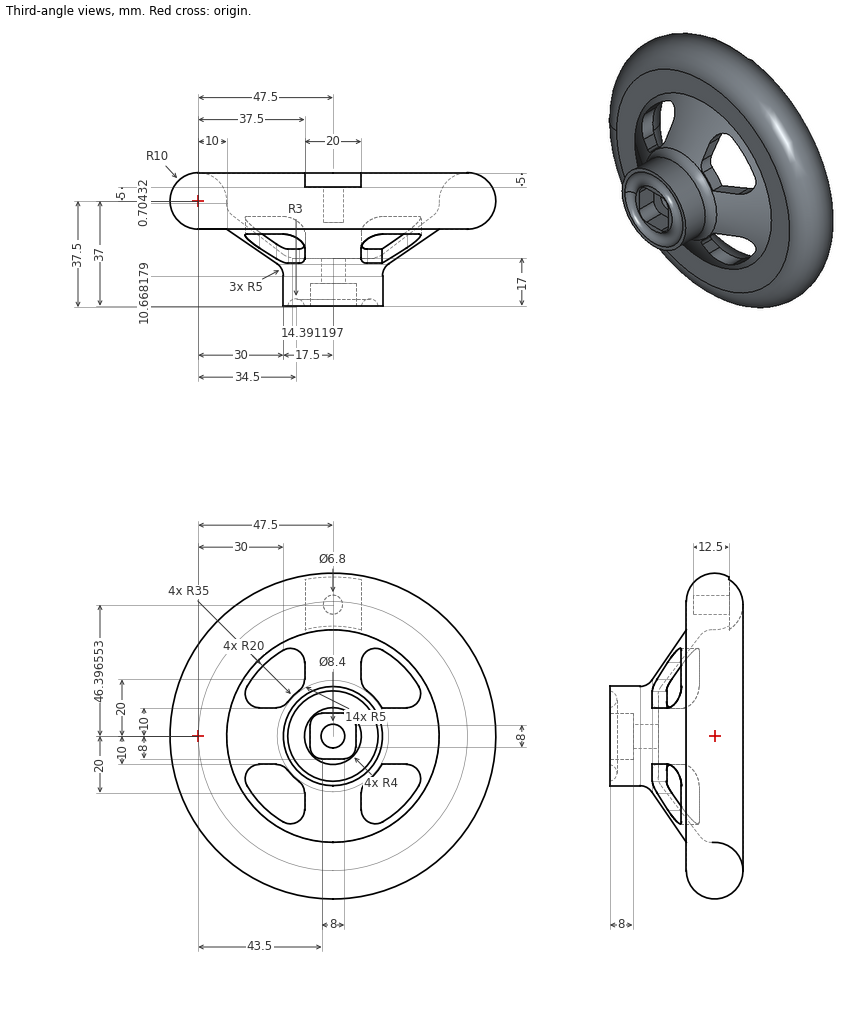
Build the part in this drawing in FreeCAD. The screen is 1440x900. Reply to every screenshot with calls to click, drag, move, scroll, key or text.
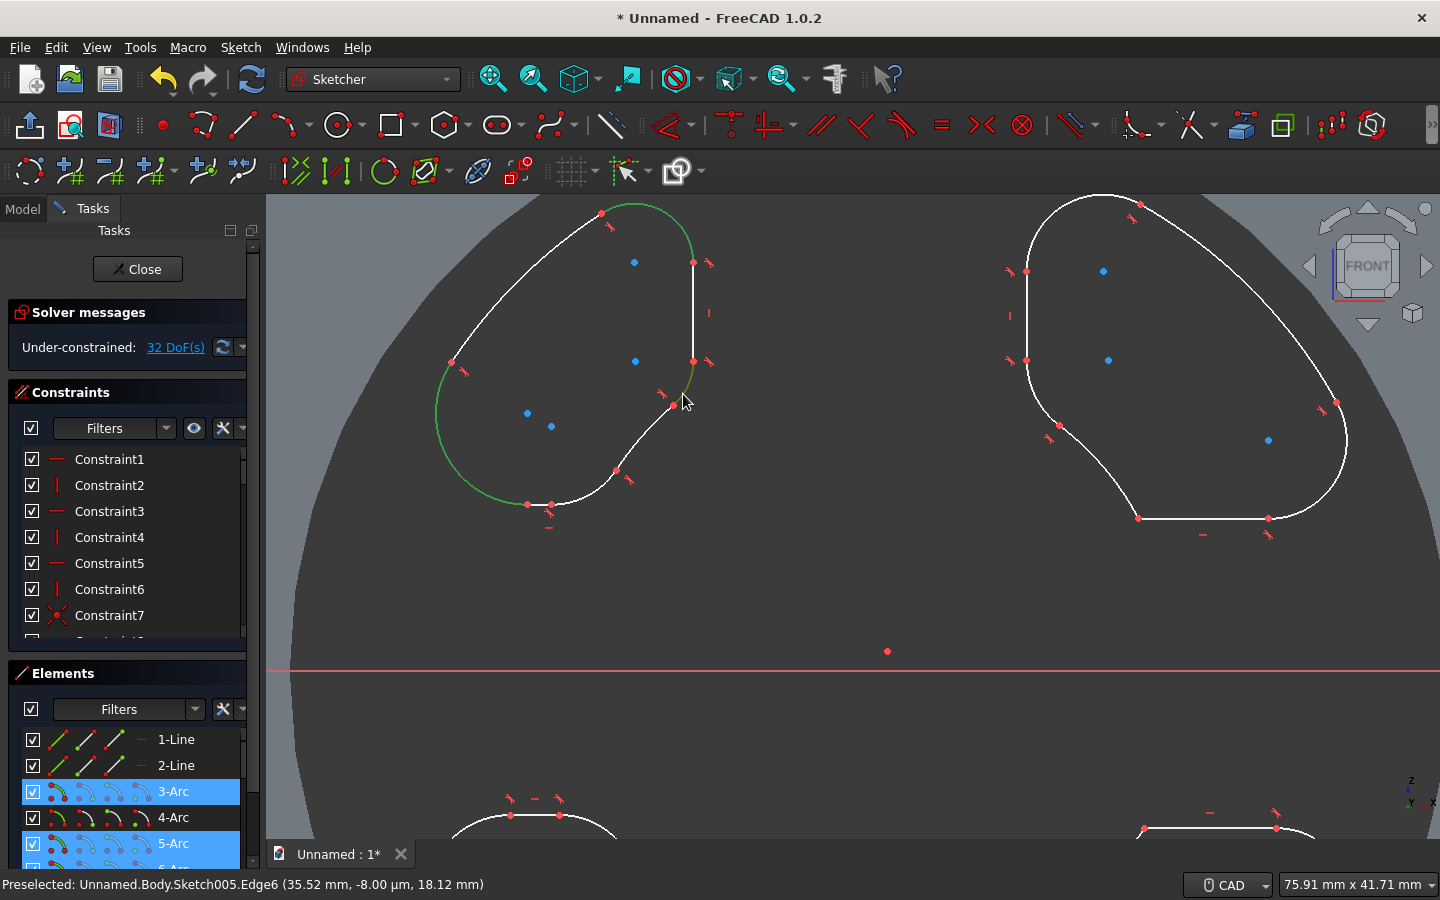
click(574, 501)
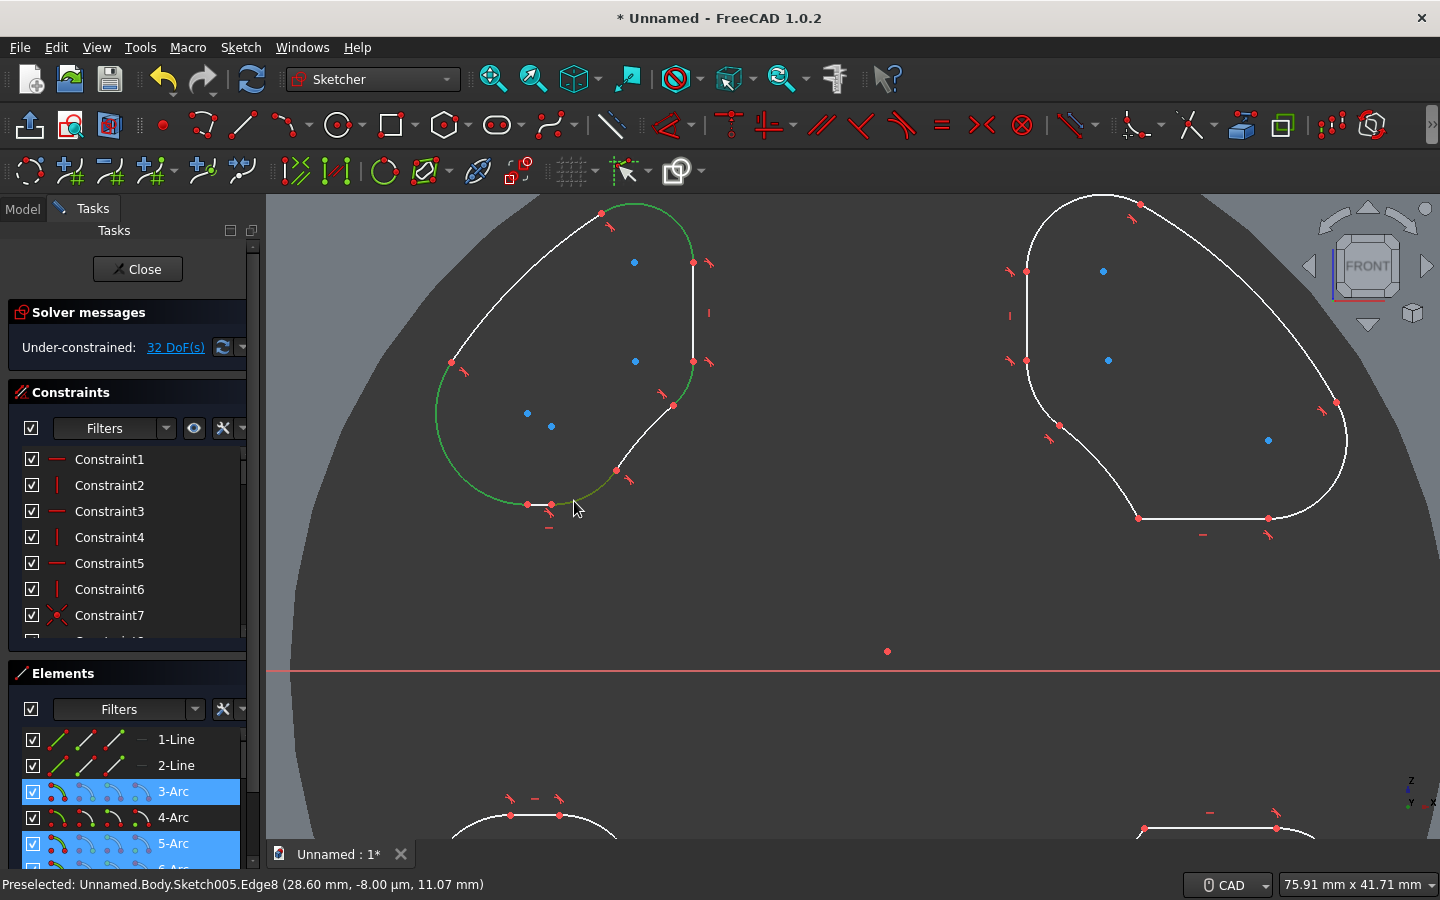
scroll(823, 390, down, 4)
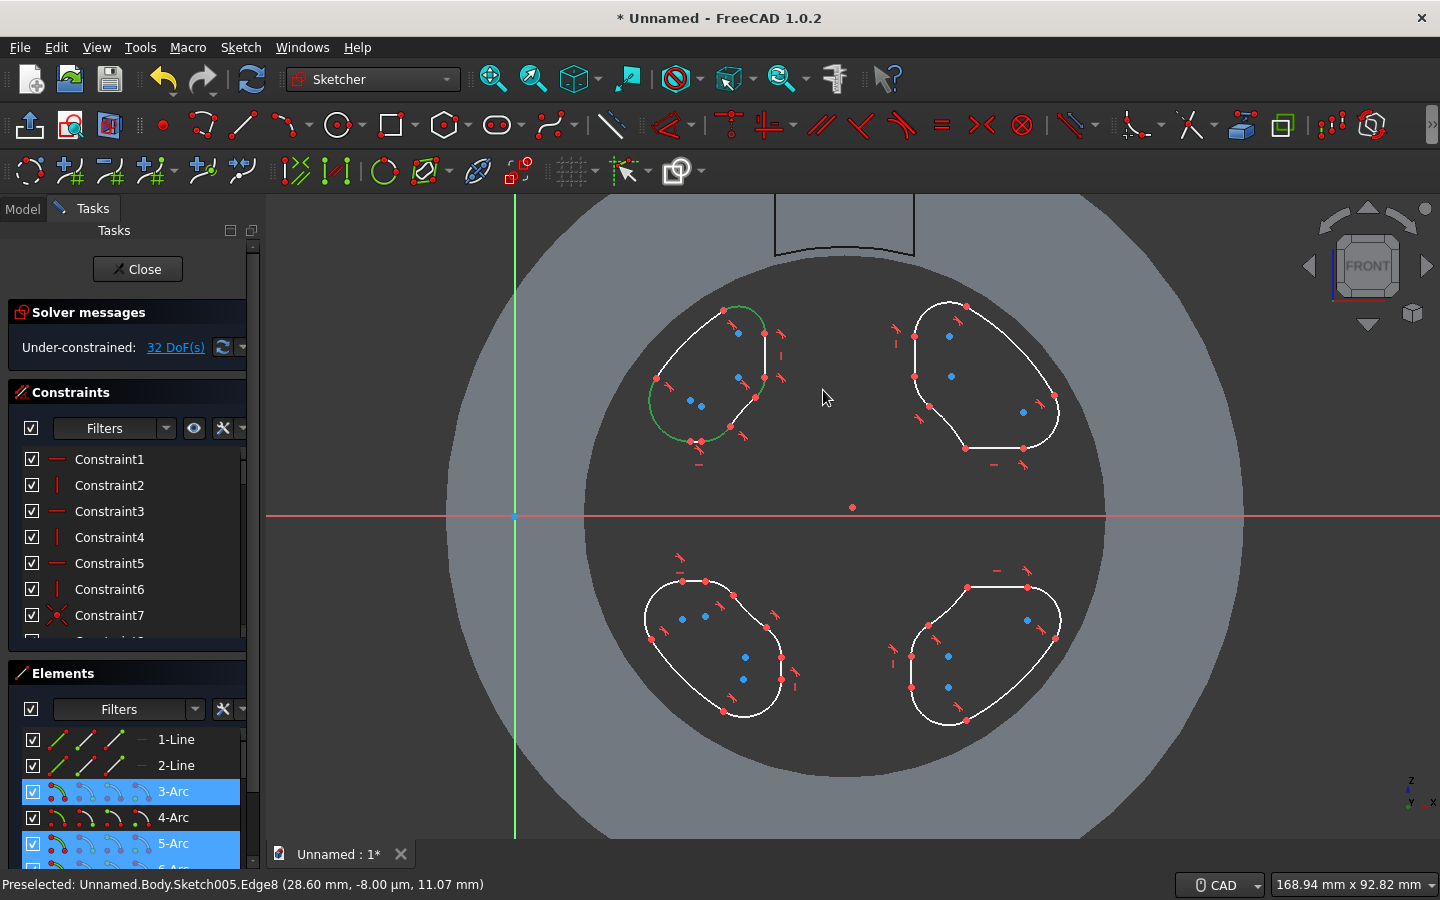
scroll(726, 588, up, 2)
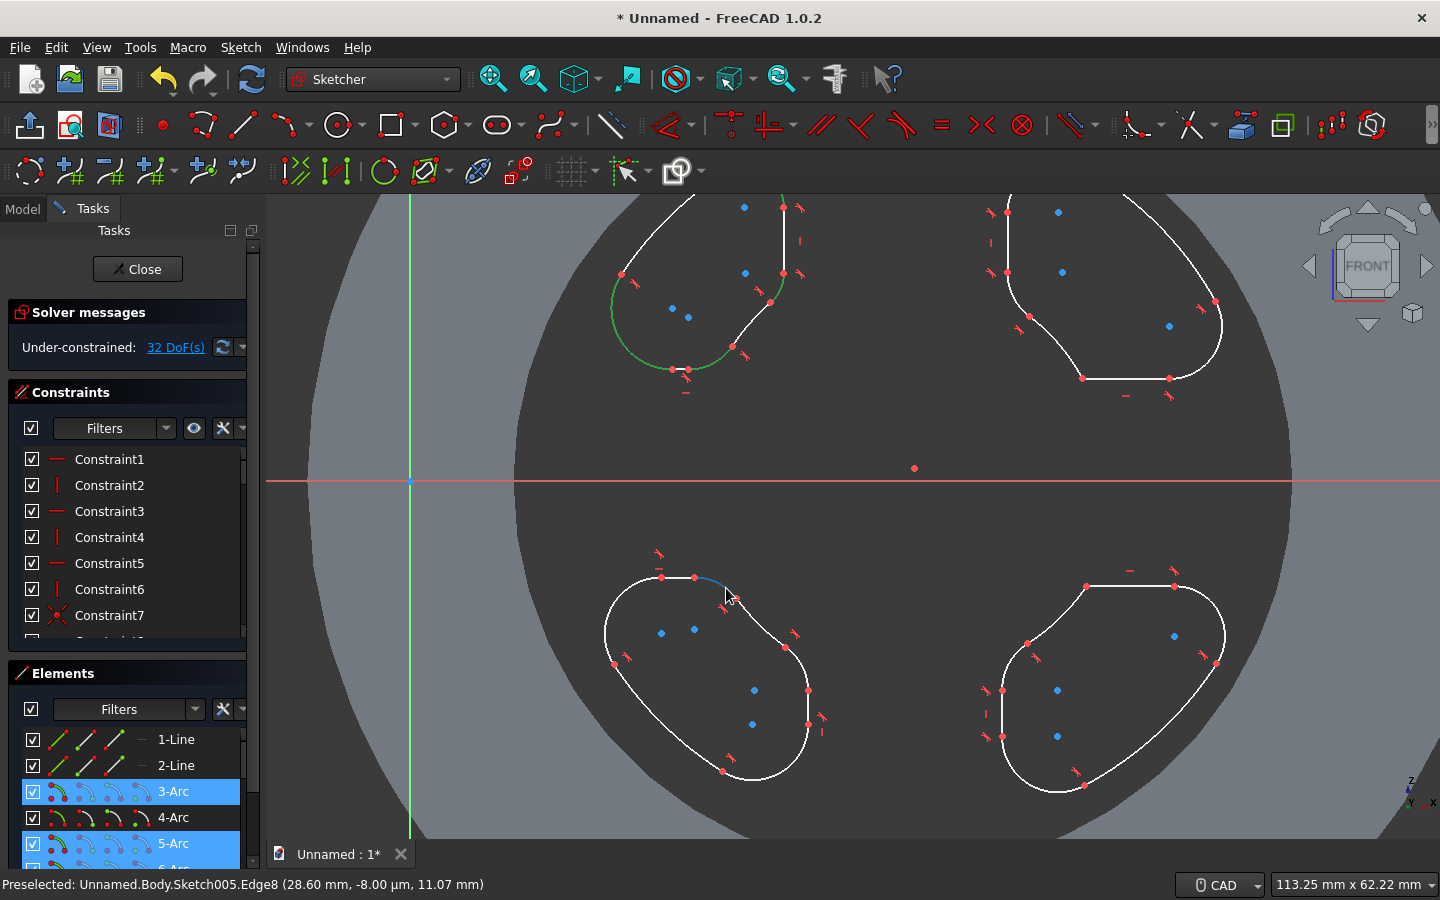
click(727, 588)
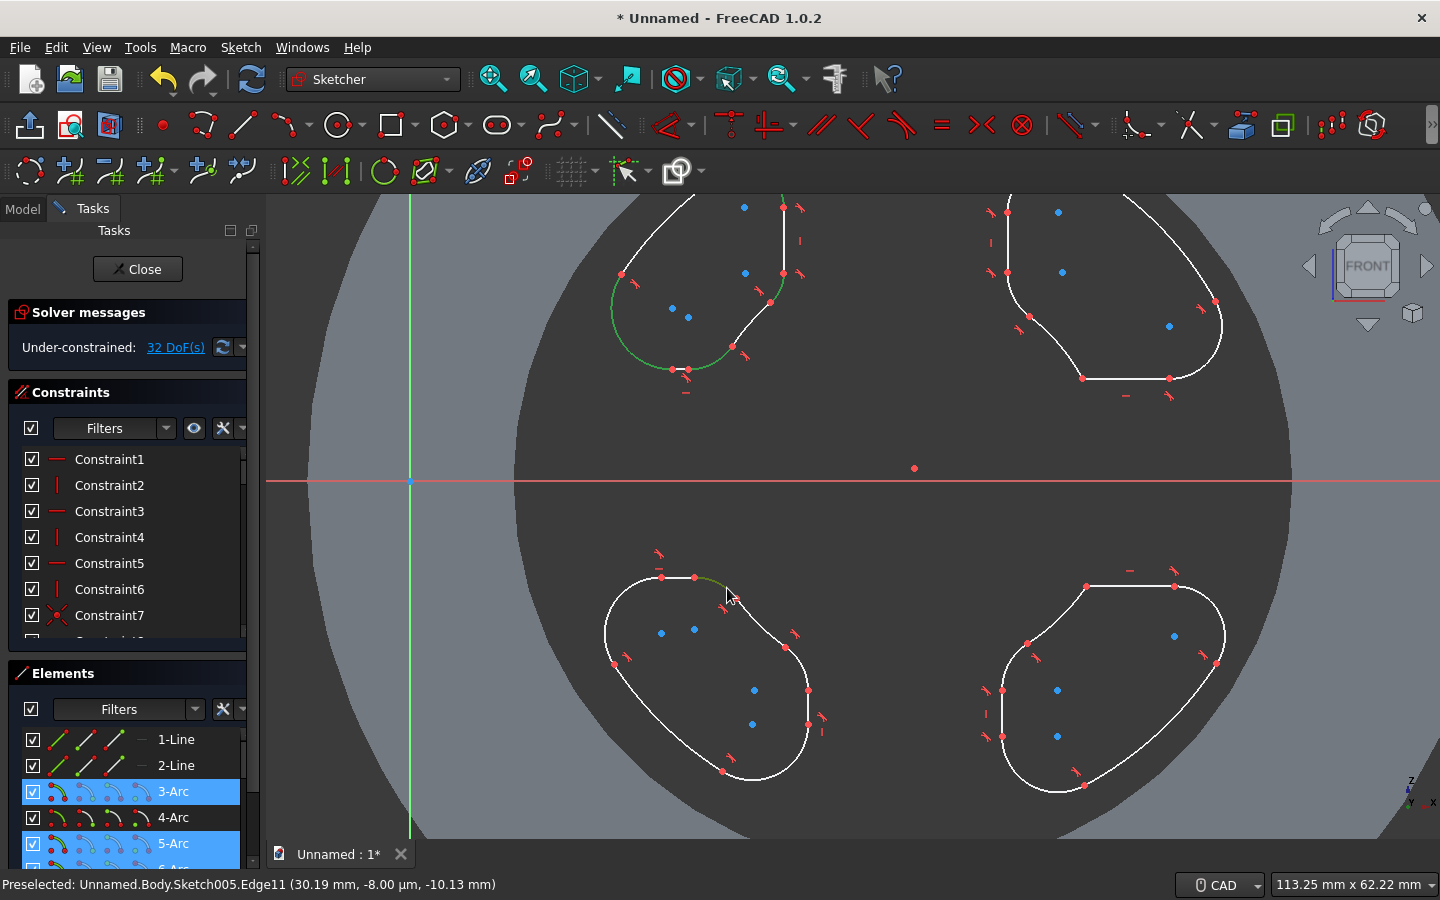
click(806, 676)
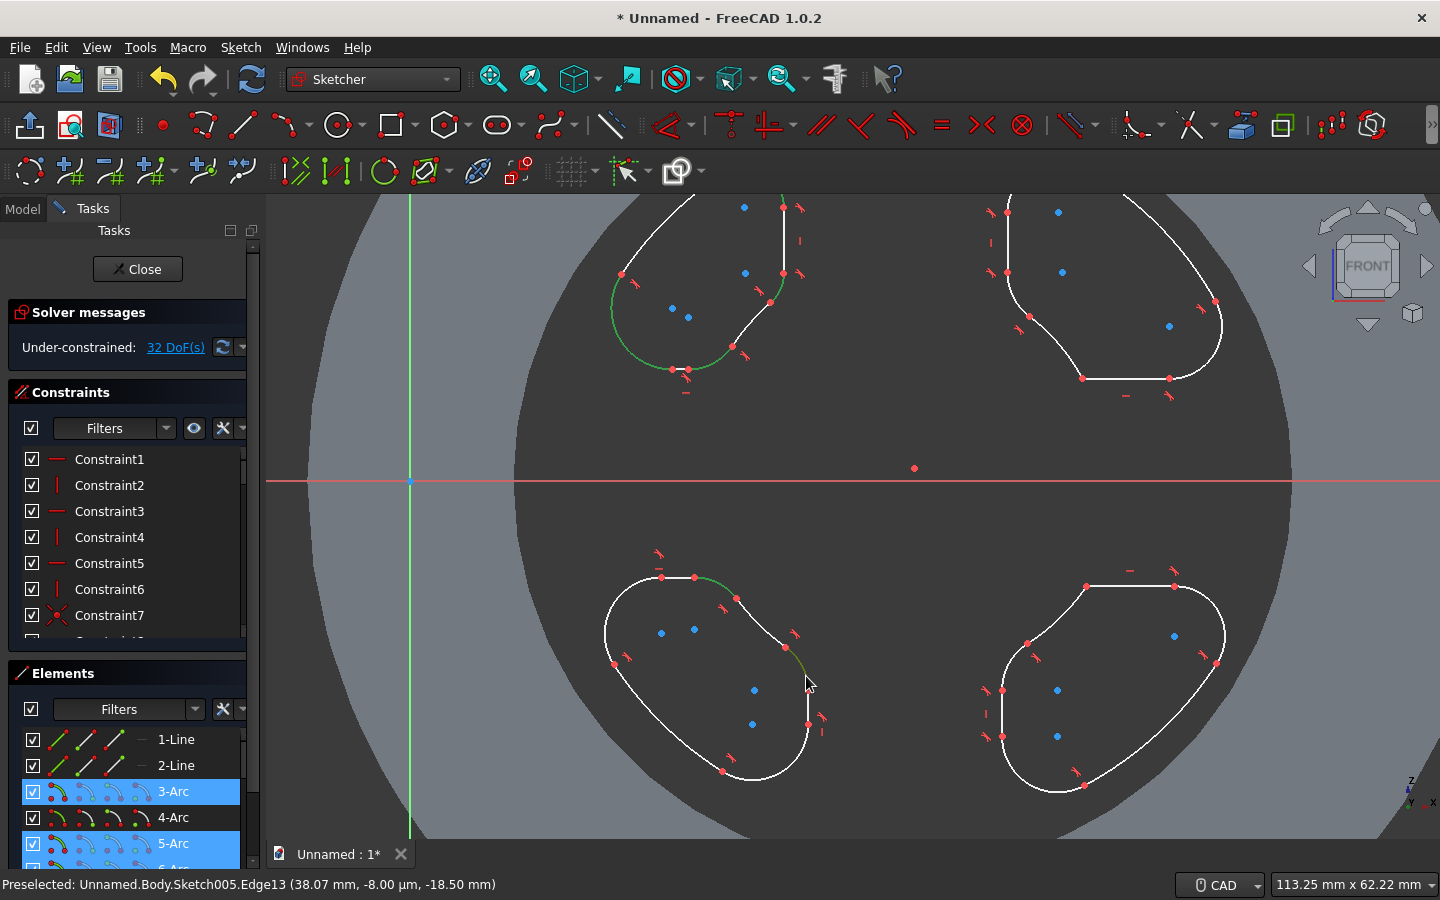
click(757, 780)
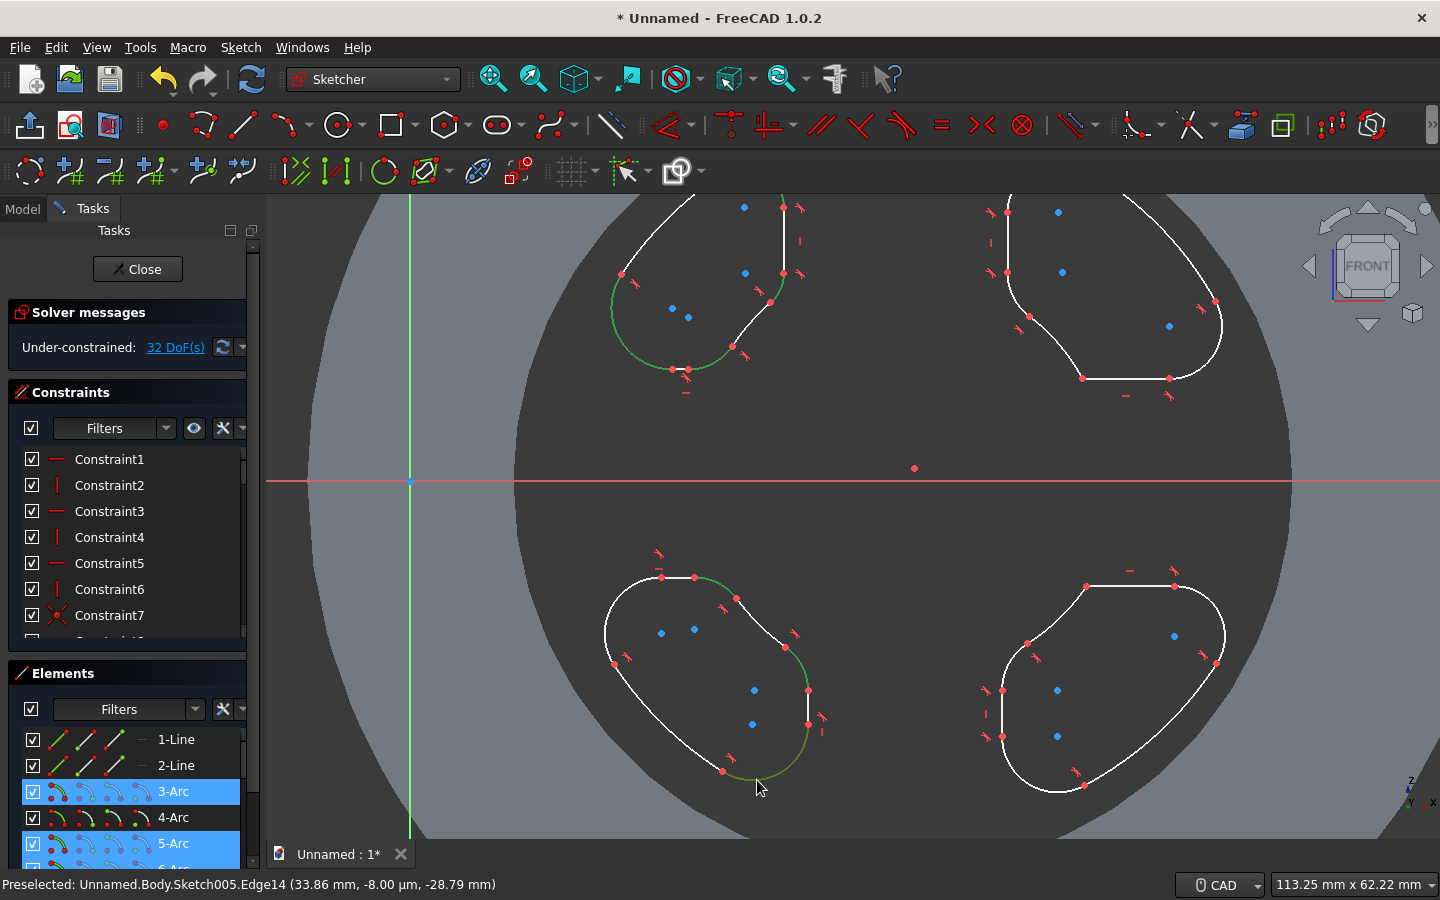
click(627, 589)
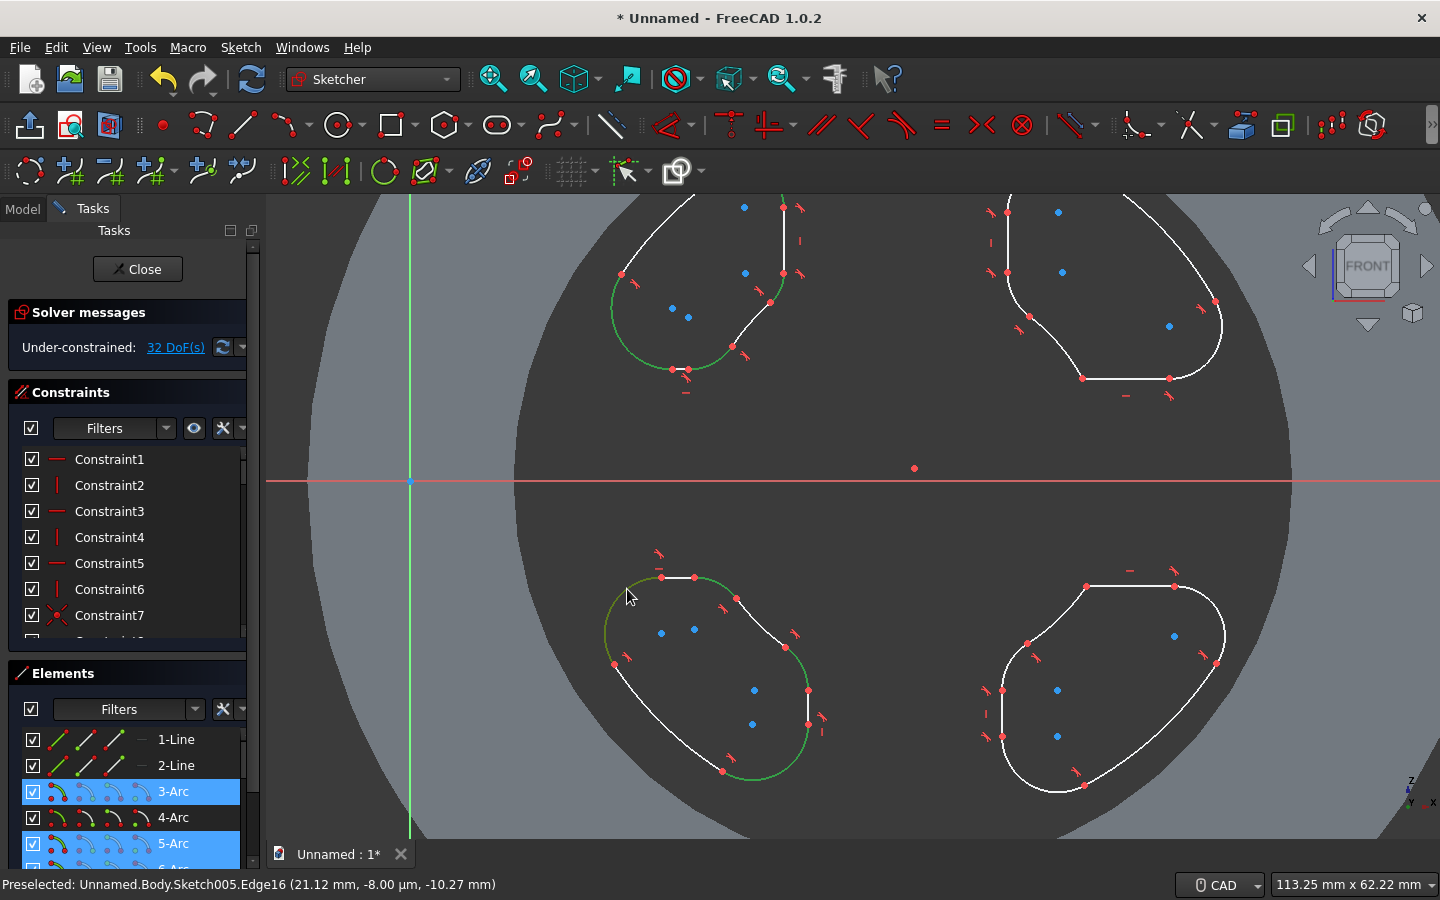
click(1225, 633)